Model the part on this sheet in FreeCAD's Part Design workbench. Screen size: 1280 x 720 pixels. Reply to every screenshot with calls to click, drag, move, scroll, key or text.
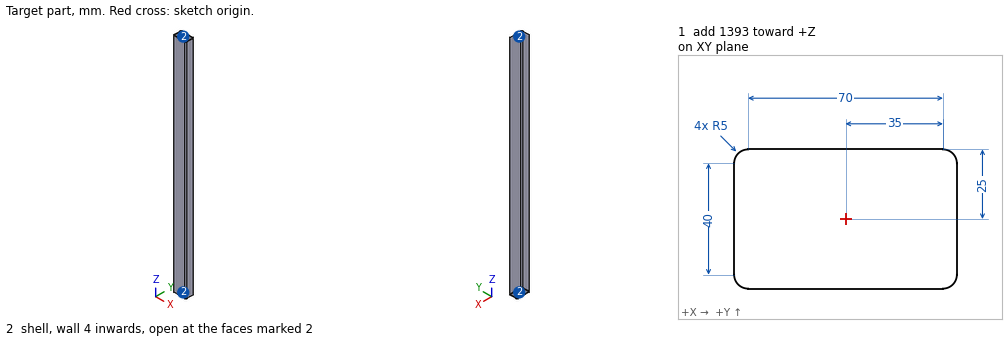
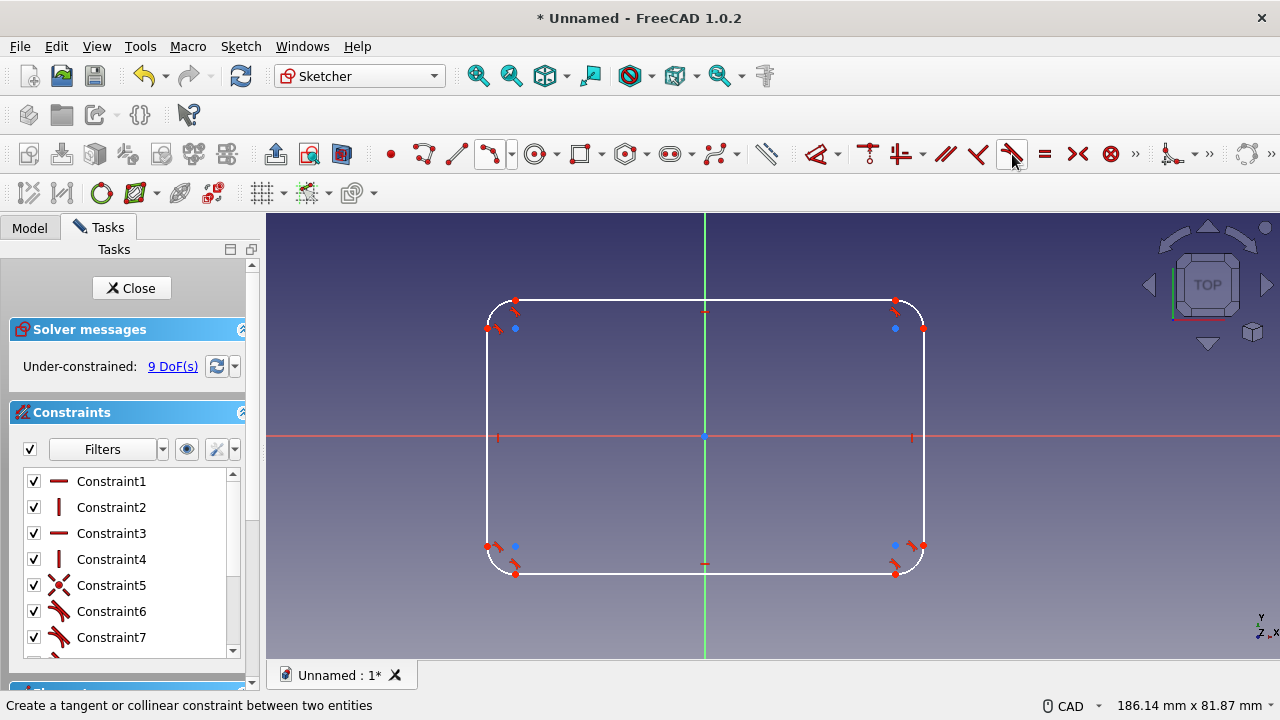
click(924, 481)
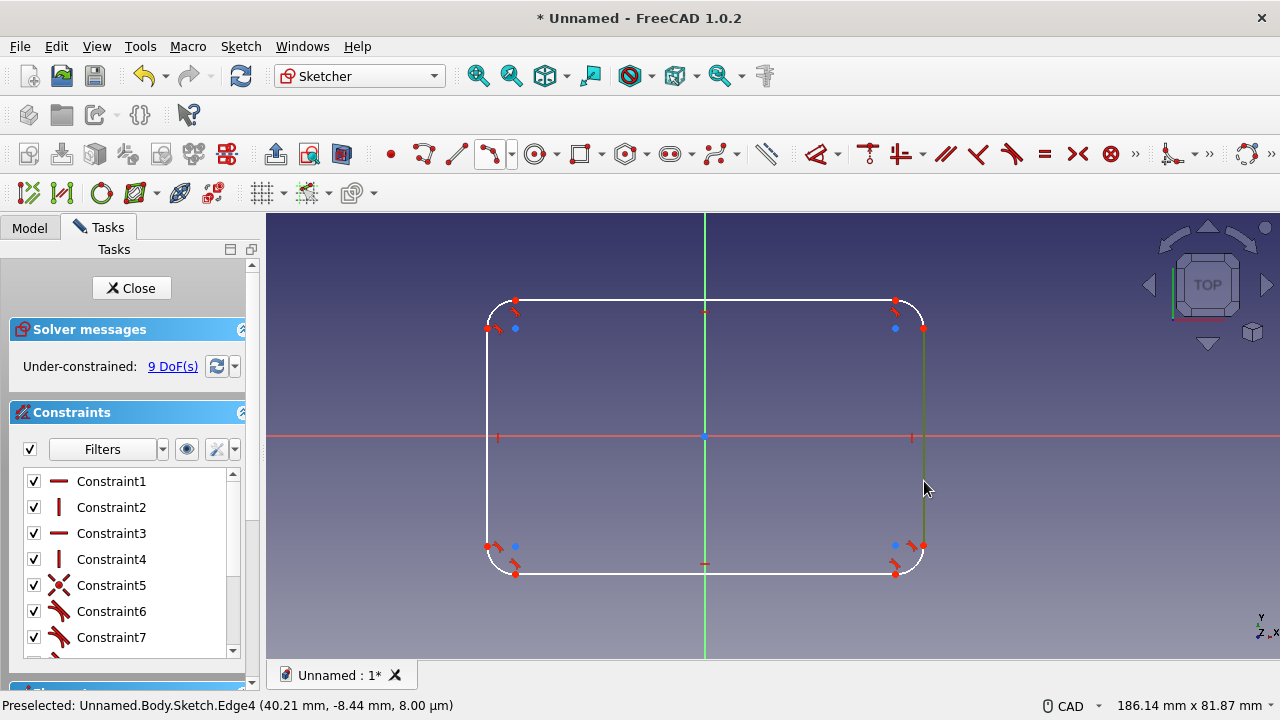
click(920, 316)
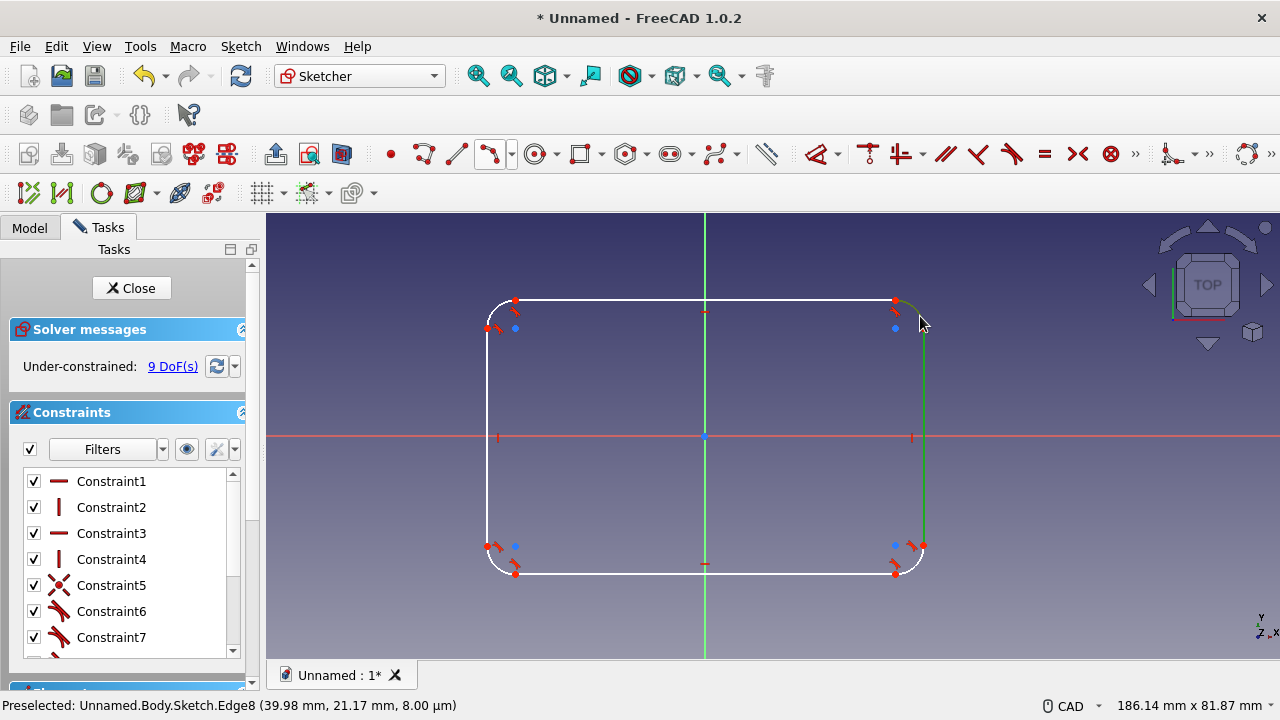
click(1012, 154)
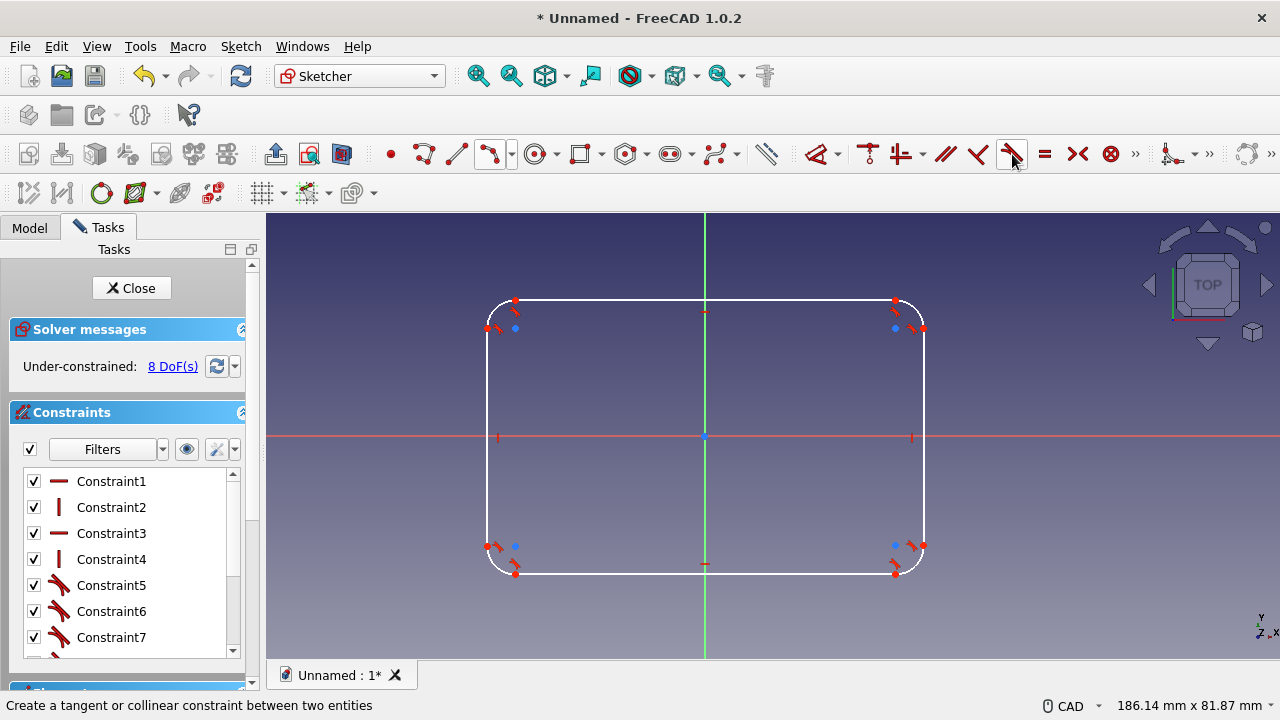
click(503, 304)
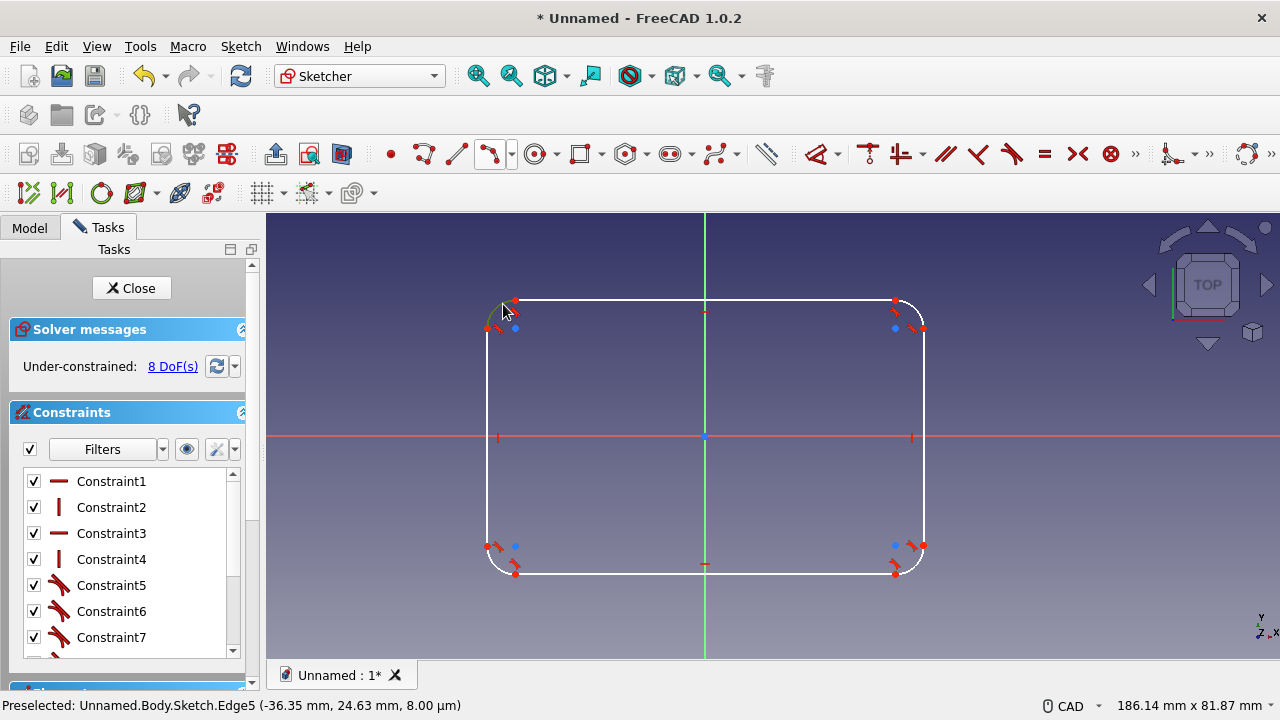
click(490, 559)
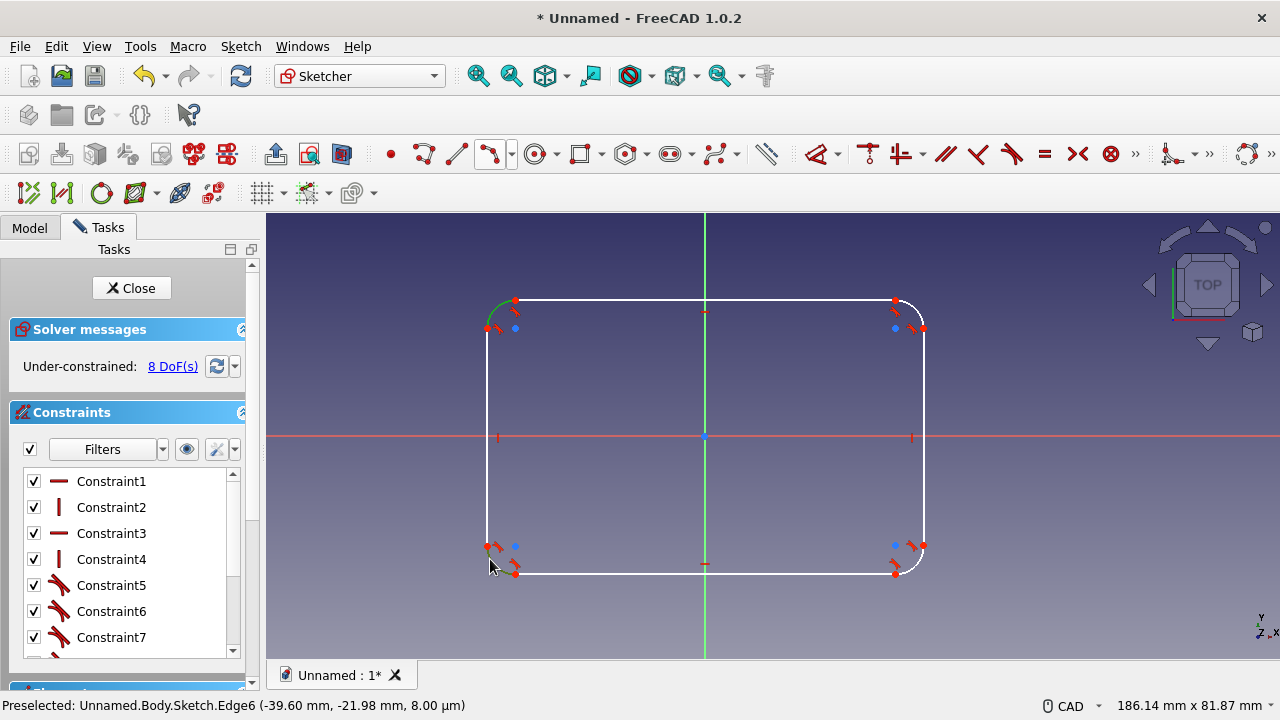
click(908, 571)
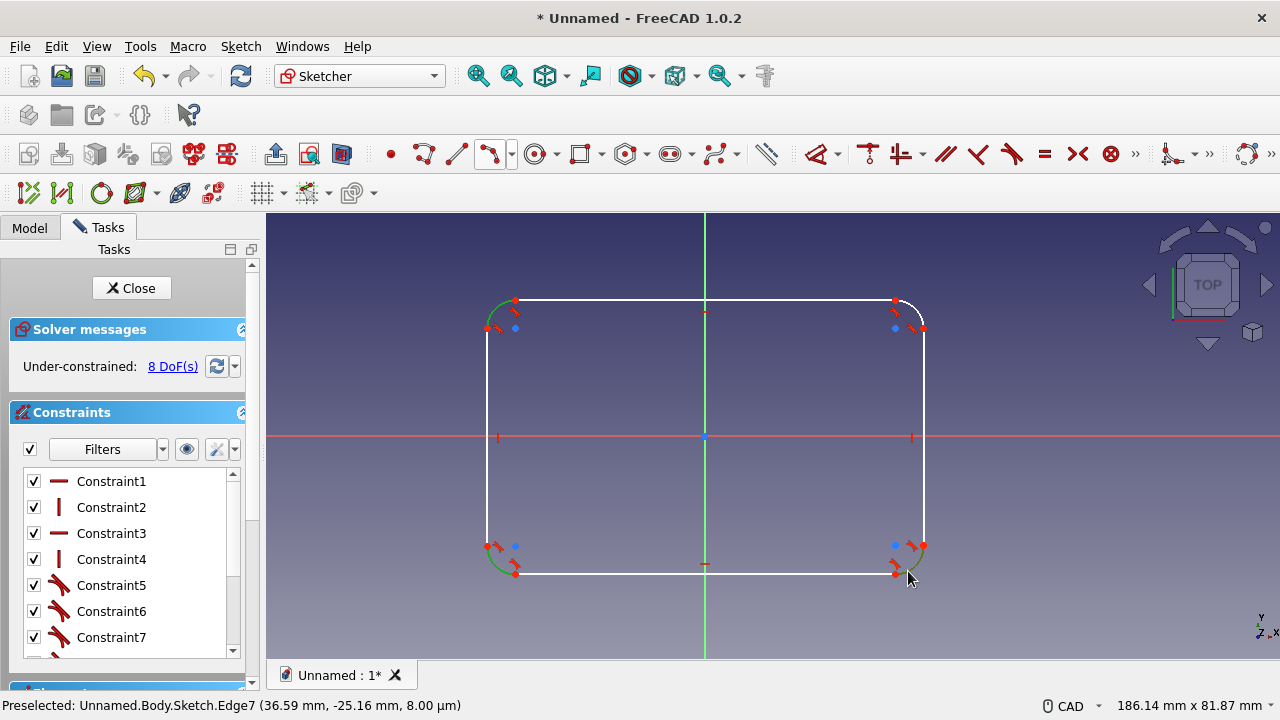
click(921, 316)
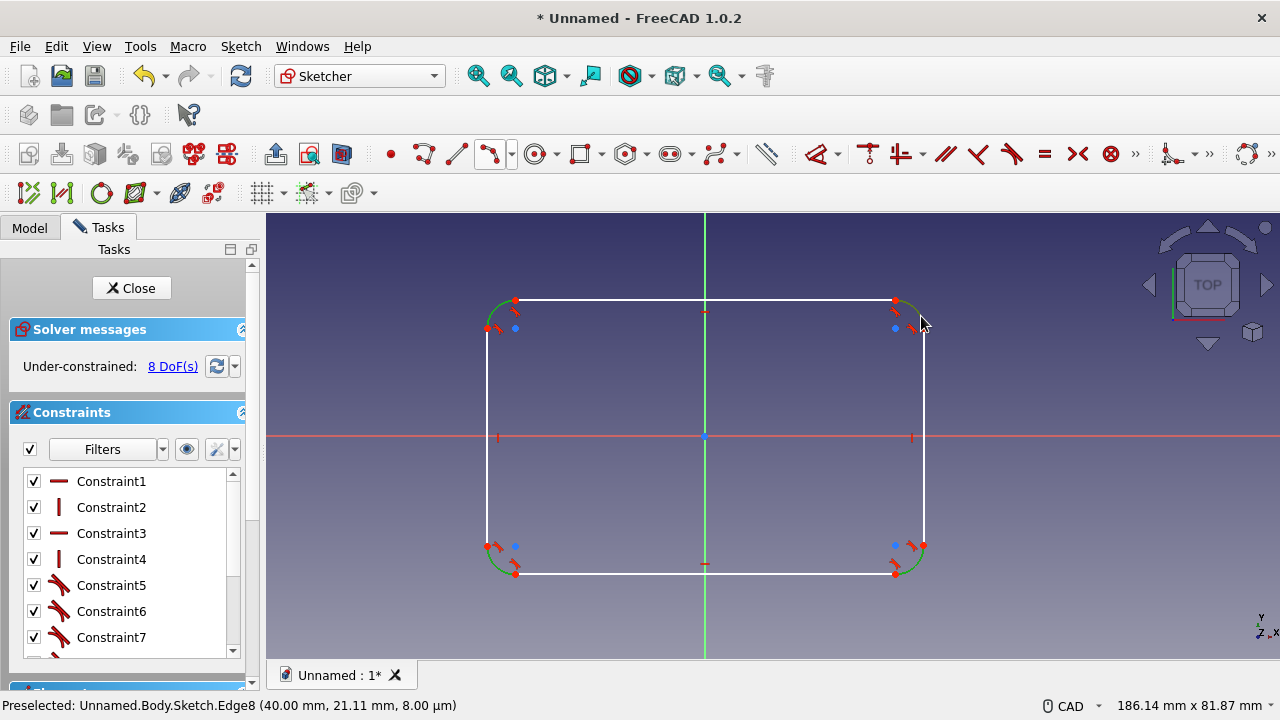
click(1045, 154)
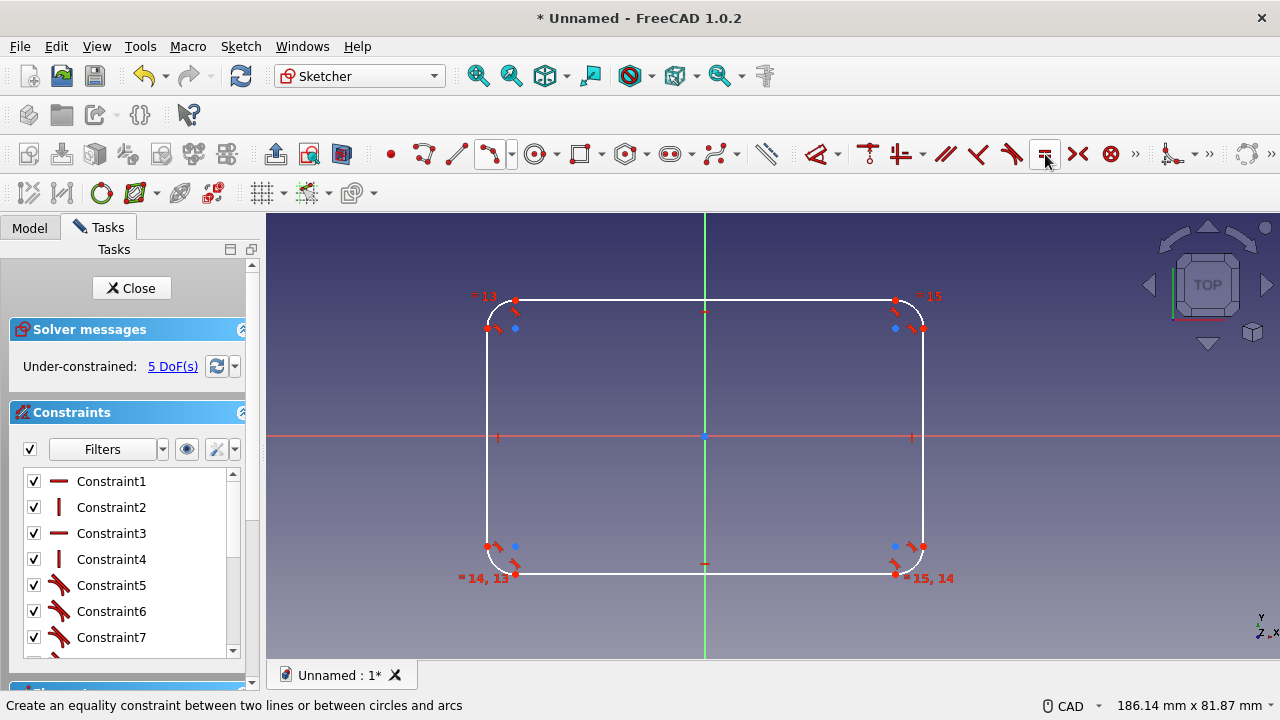
scroll(503, 304, up, 2)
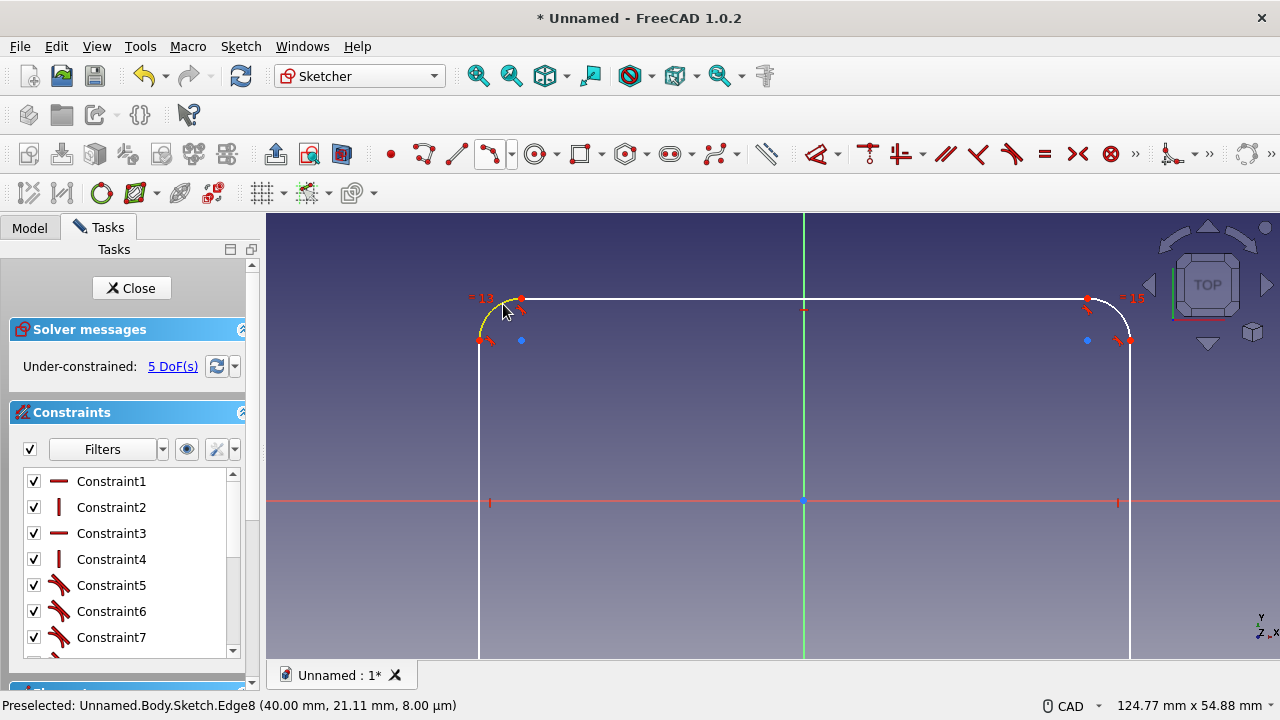
click(502, 303)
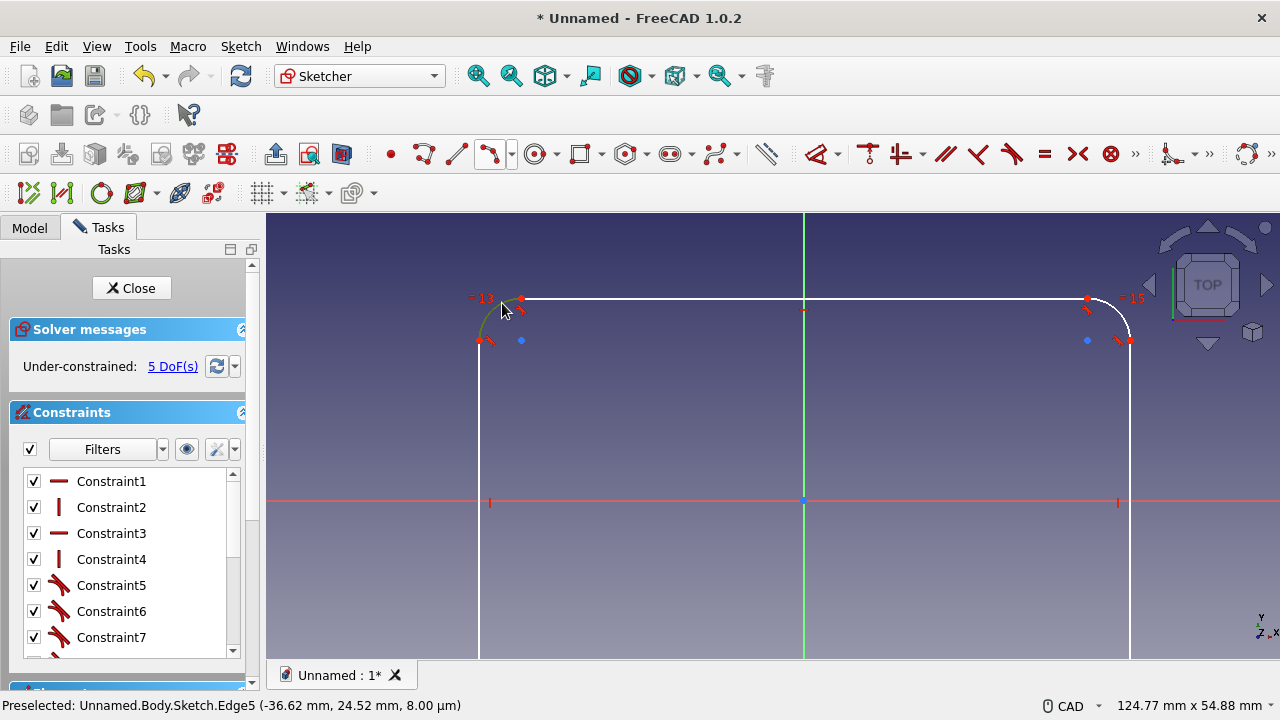
click(838, 154)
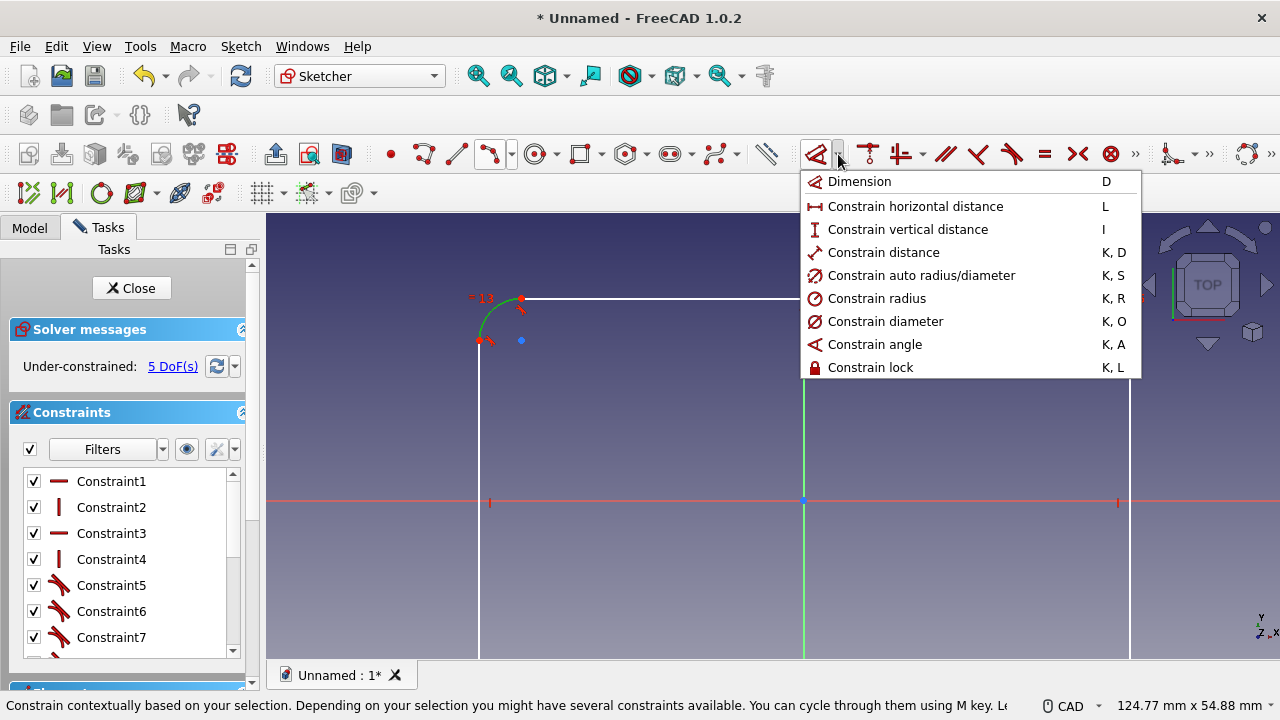
click(971, 298)